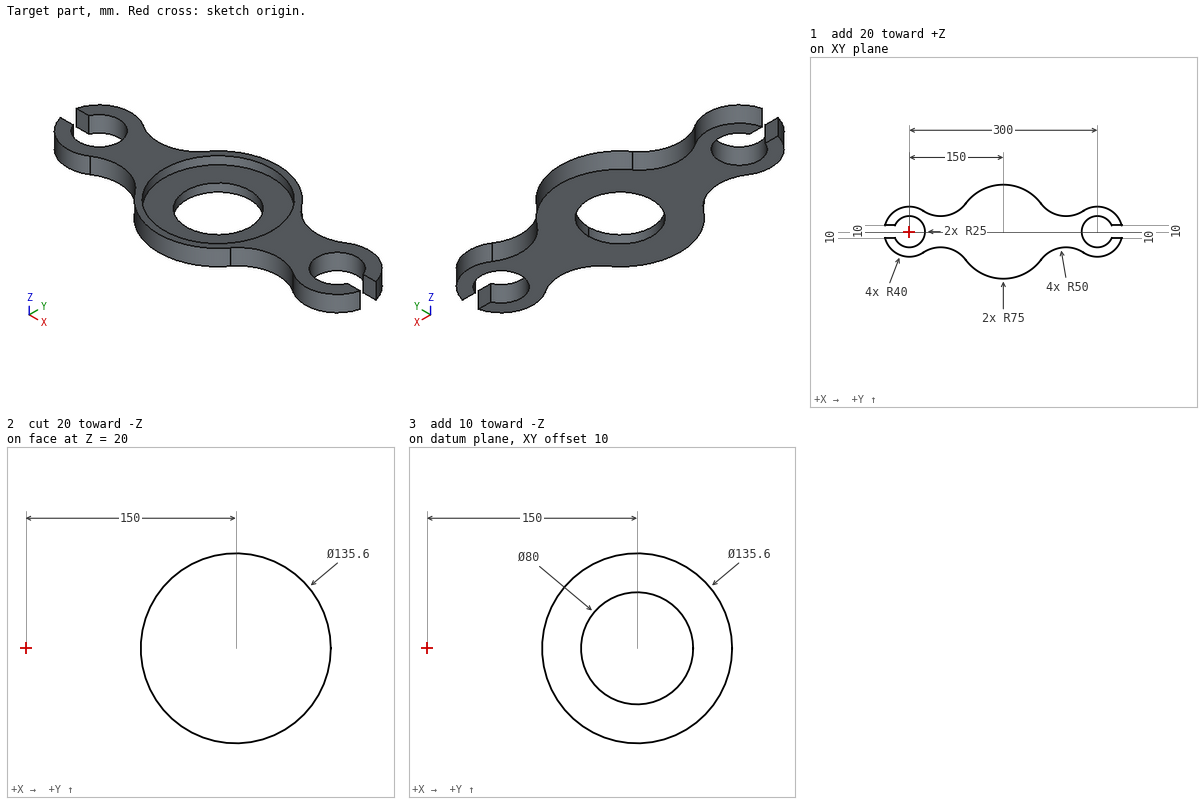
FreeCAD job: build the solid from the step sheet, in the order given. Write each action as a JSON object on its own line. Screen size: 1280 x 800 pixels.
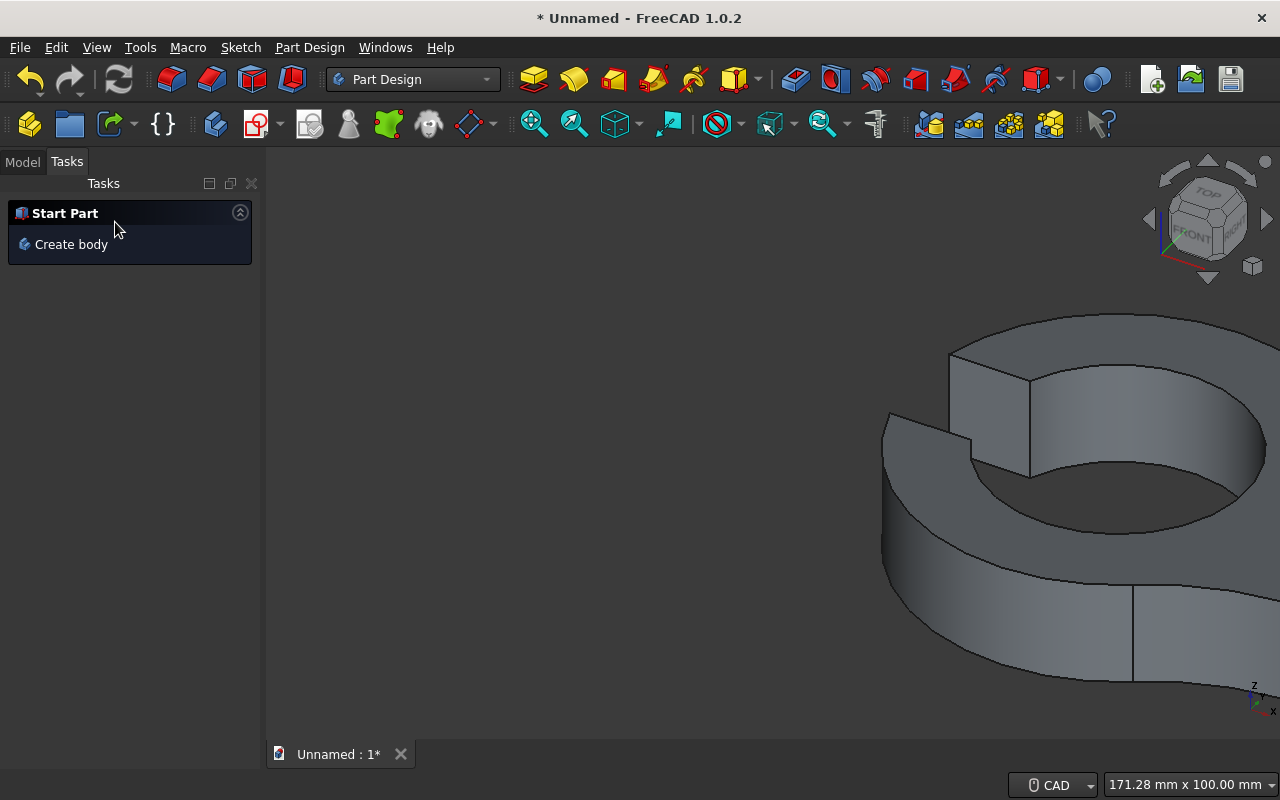
{"action": "left_click", "coordinate": [536, 124]}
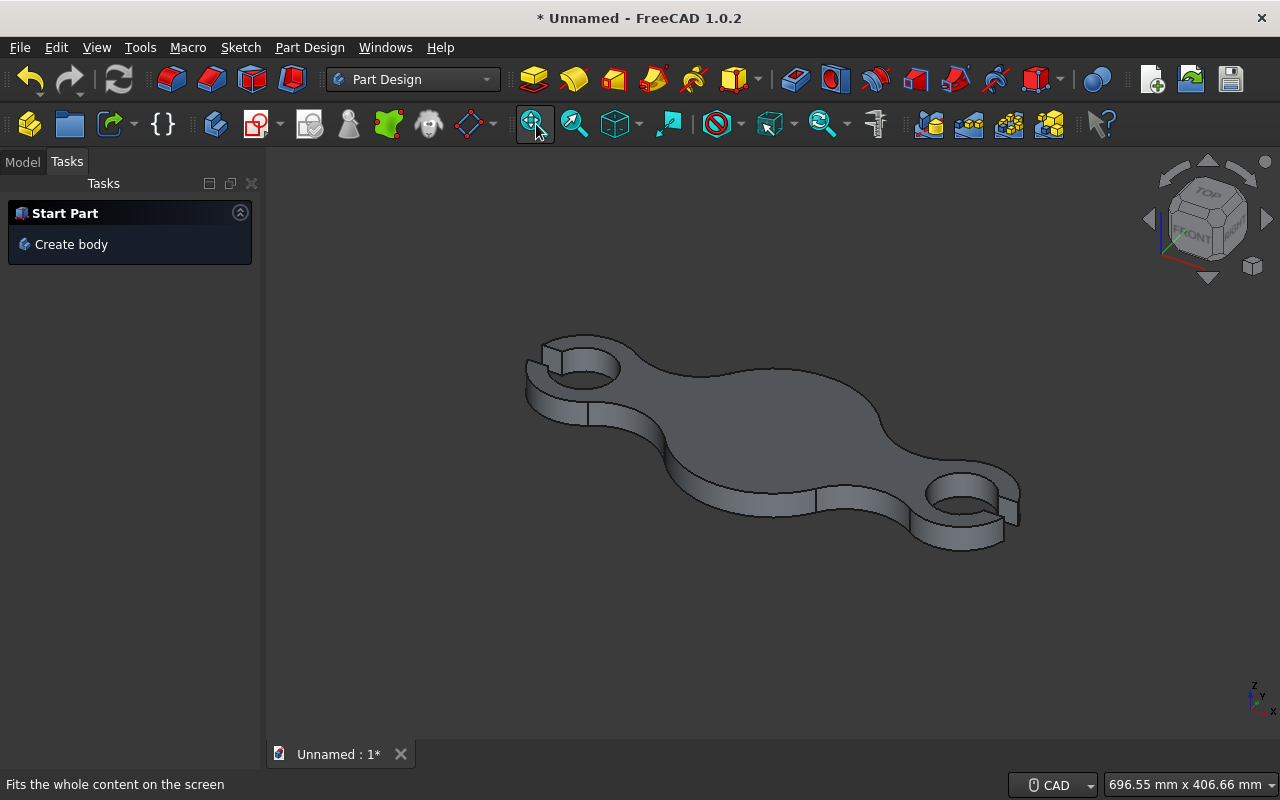
{"action": "left_click", "coordinate": [773, 430]}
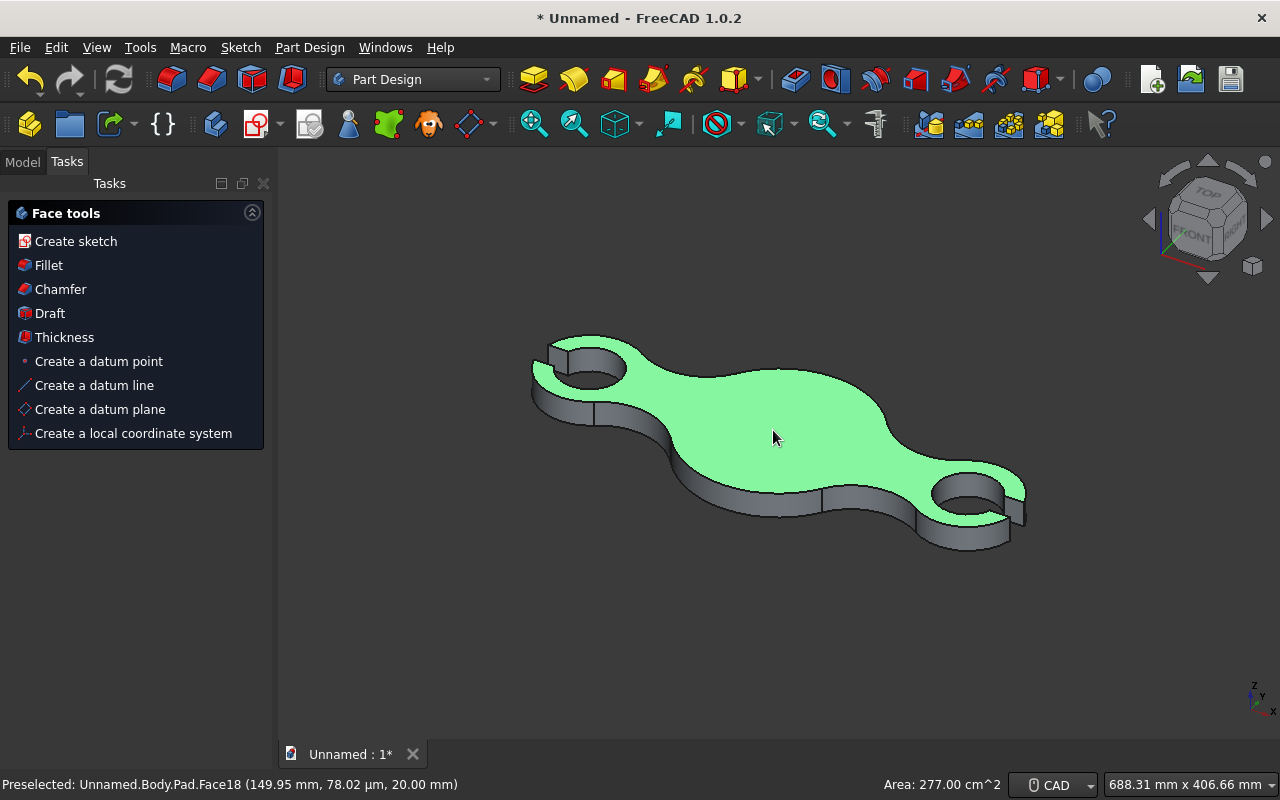
{"action": "left_click", "coordinate": [256, 124]}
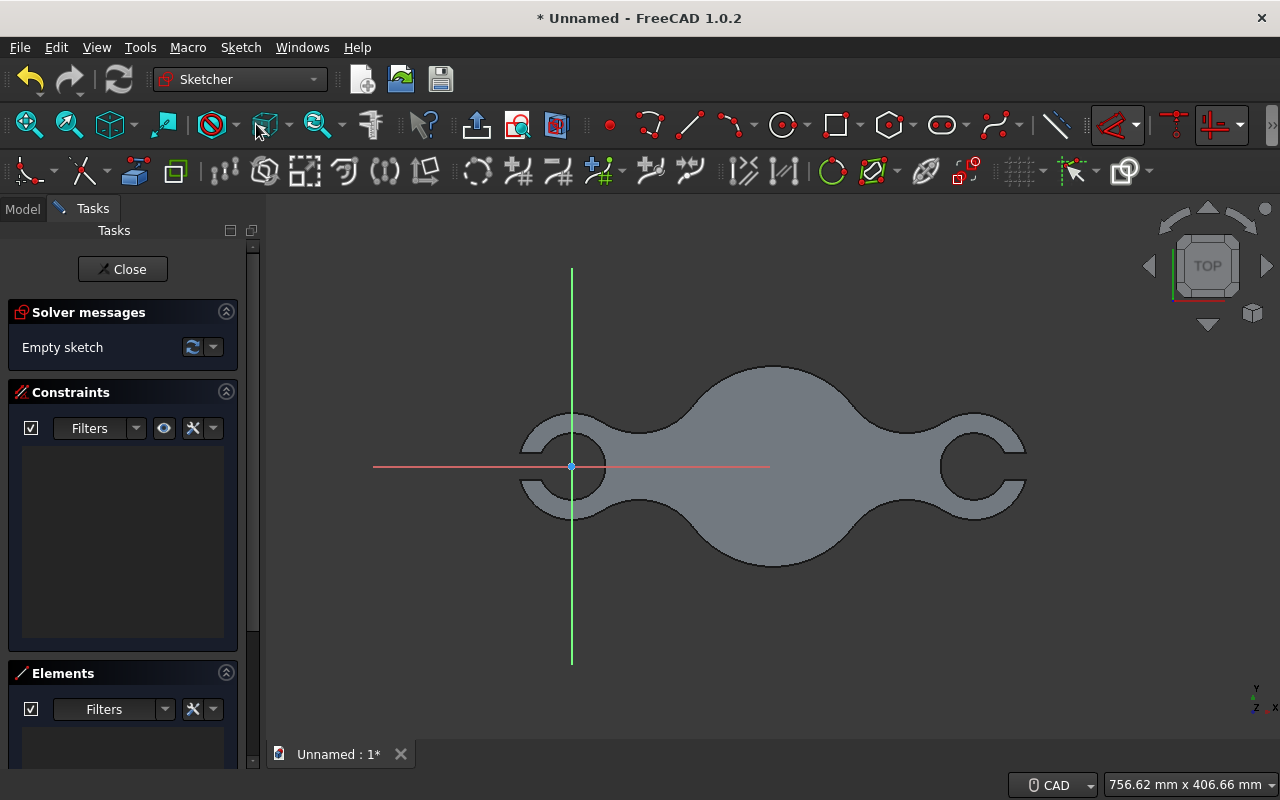
{"action": "scroll", "coordinate": [734, 466], "scroll_direction": "up", "scroll_amount": 3}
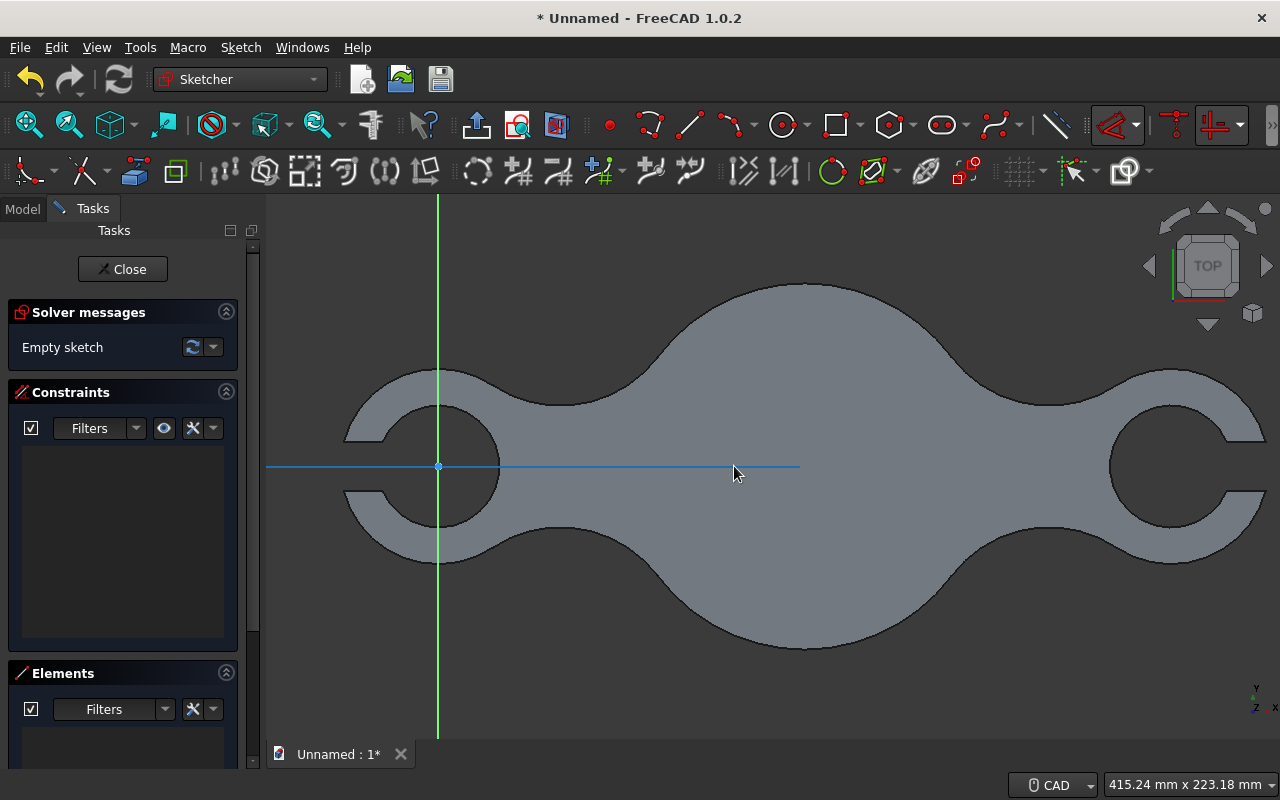
{"action": "left_click", "coordinate": [784, 126]}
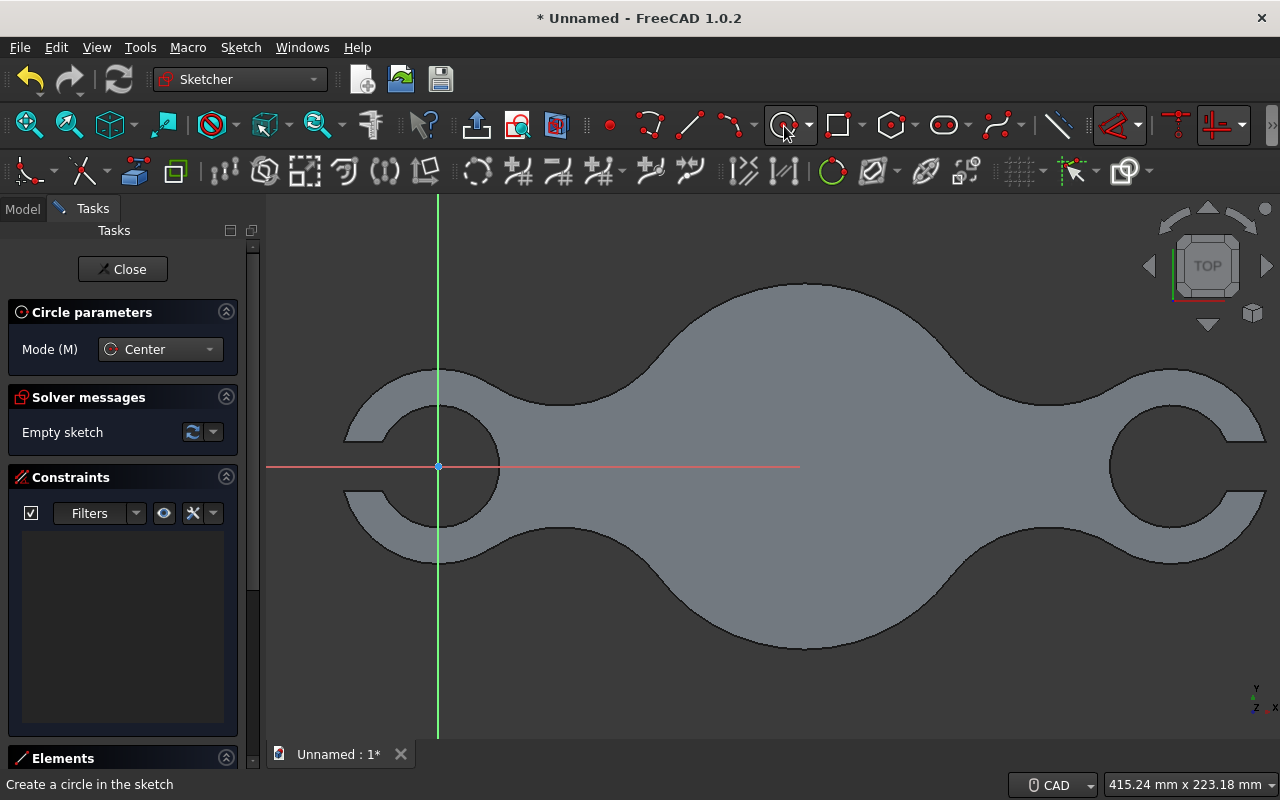
{"action": "left_click", "coordinate": [805, 466]}
{"action": "mouse_move", "coordinate": [922, 349]}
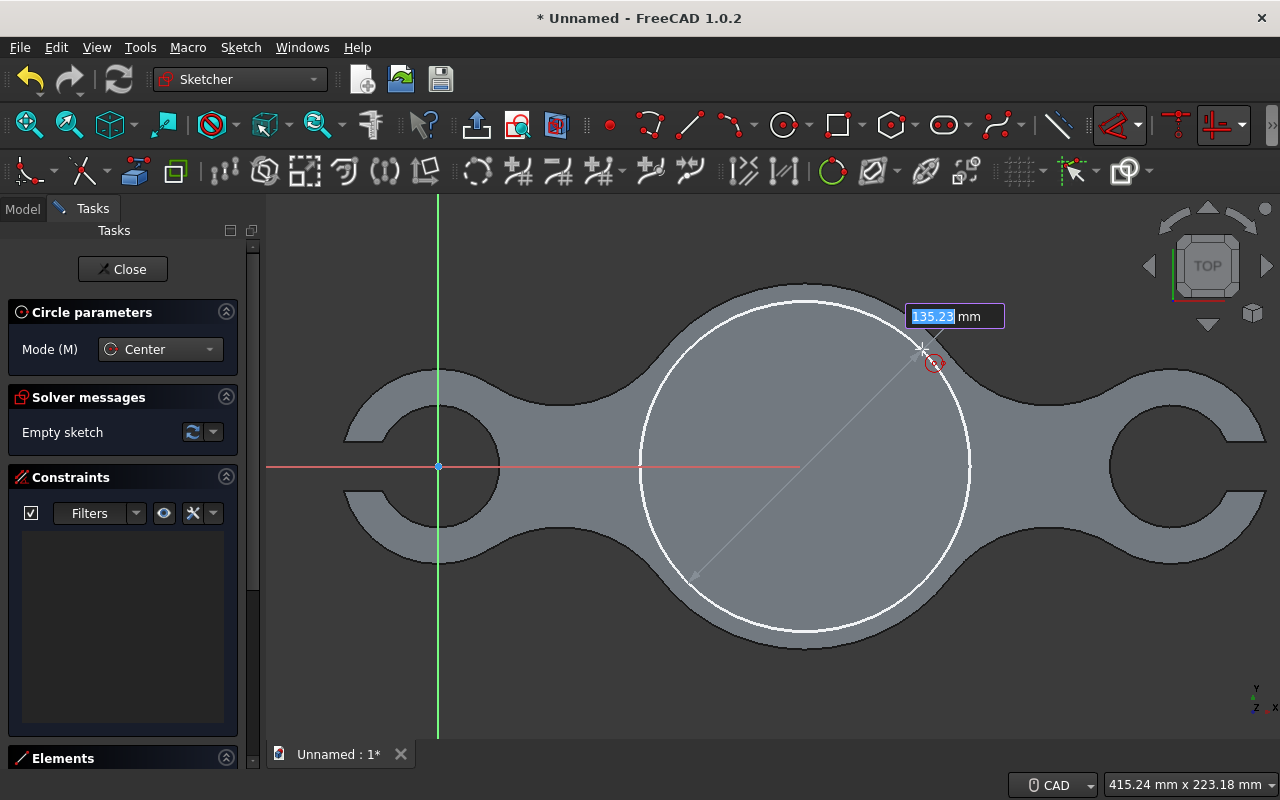
{"action": "type", "text": "135.6"}
{"action": "key", "text": "Return"}
{"action": "key", "text": "Escape"}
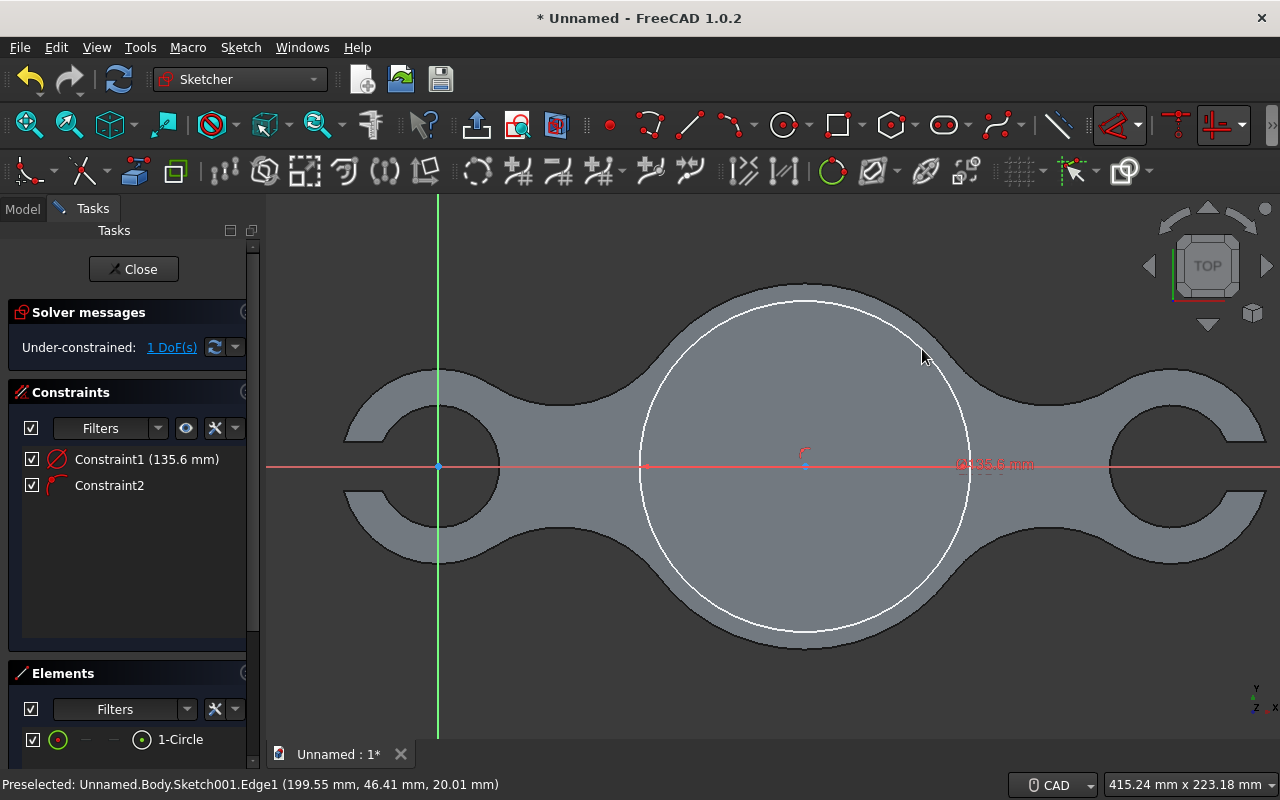
{"action": "left_click", "coordinate": [805, 466]}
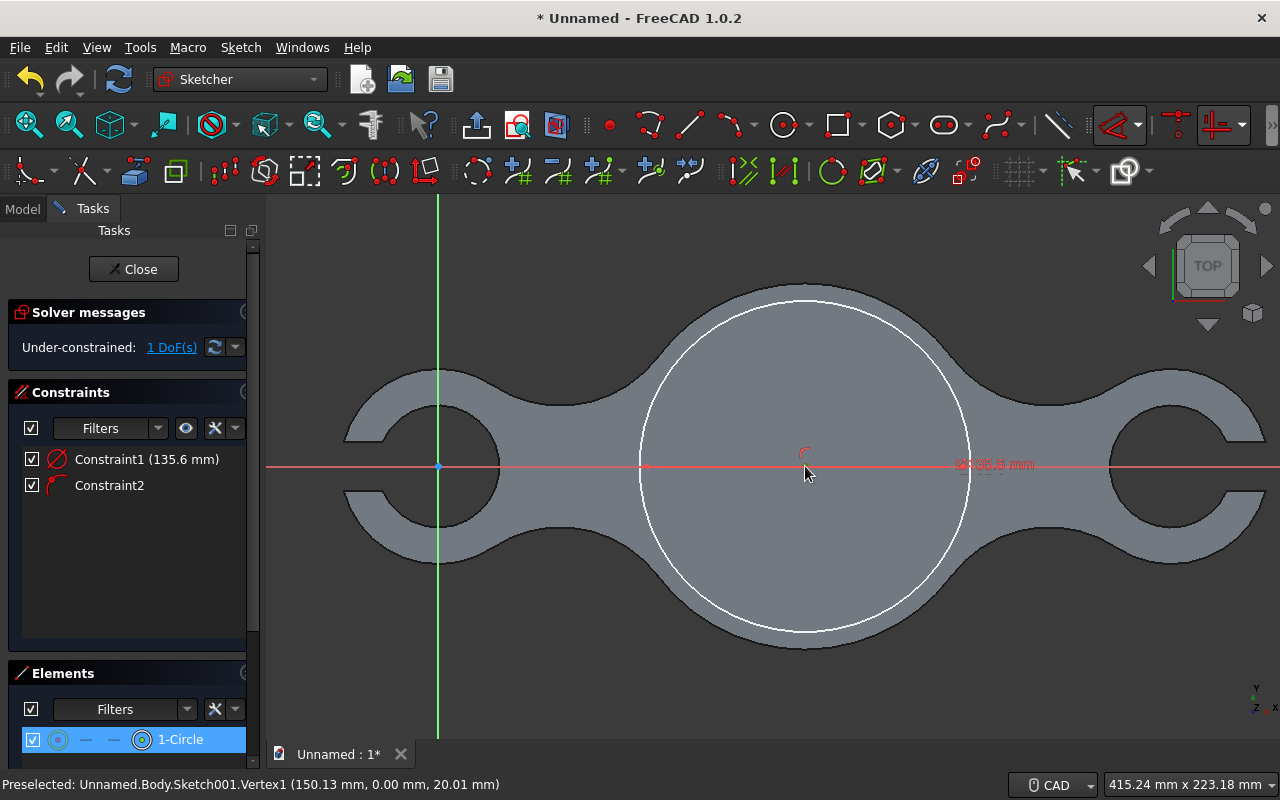
{"action": "left_click", "coordinate": [1140, 126]}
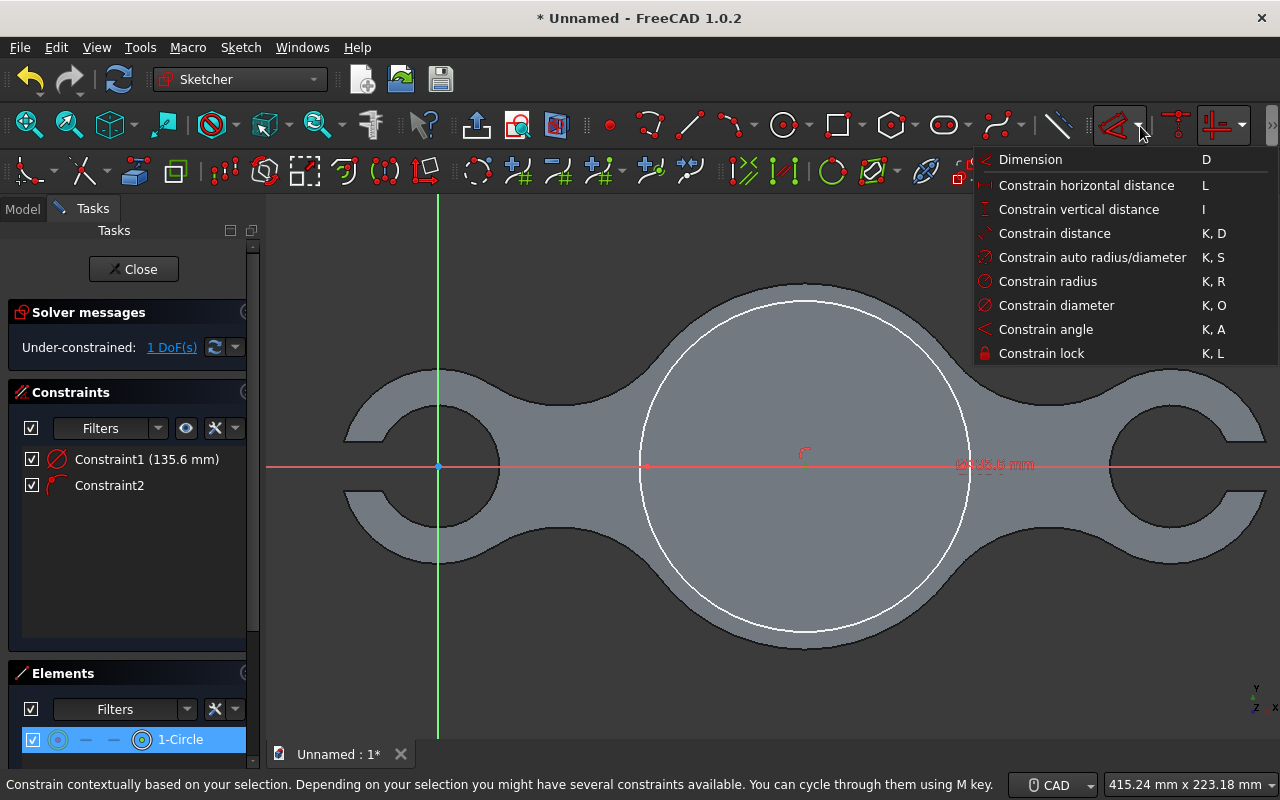
{"action": "left_click", "coordinate": [1126, 185]}